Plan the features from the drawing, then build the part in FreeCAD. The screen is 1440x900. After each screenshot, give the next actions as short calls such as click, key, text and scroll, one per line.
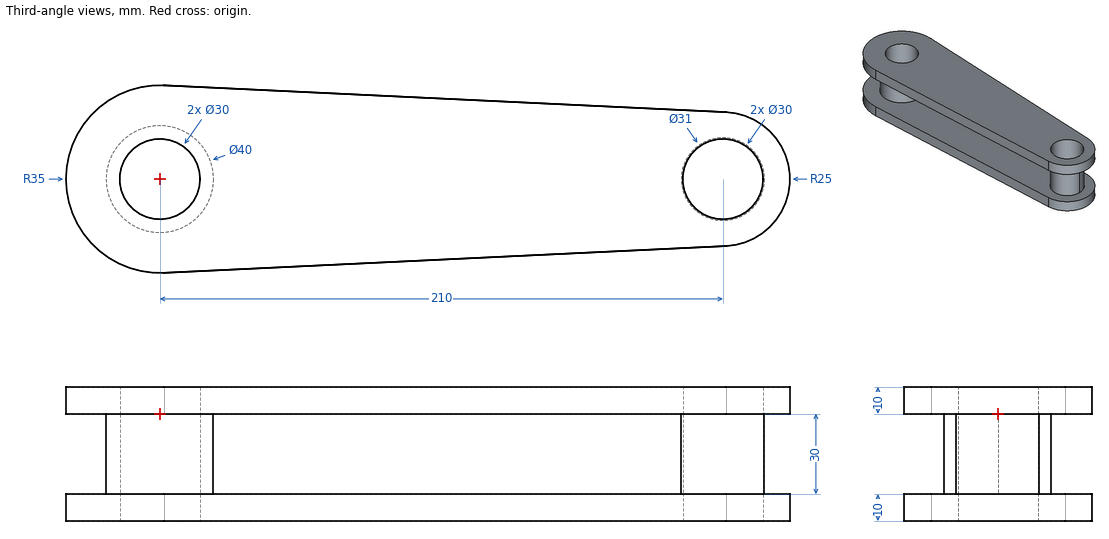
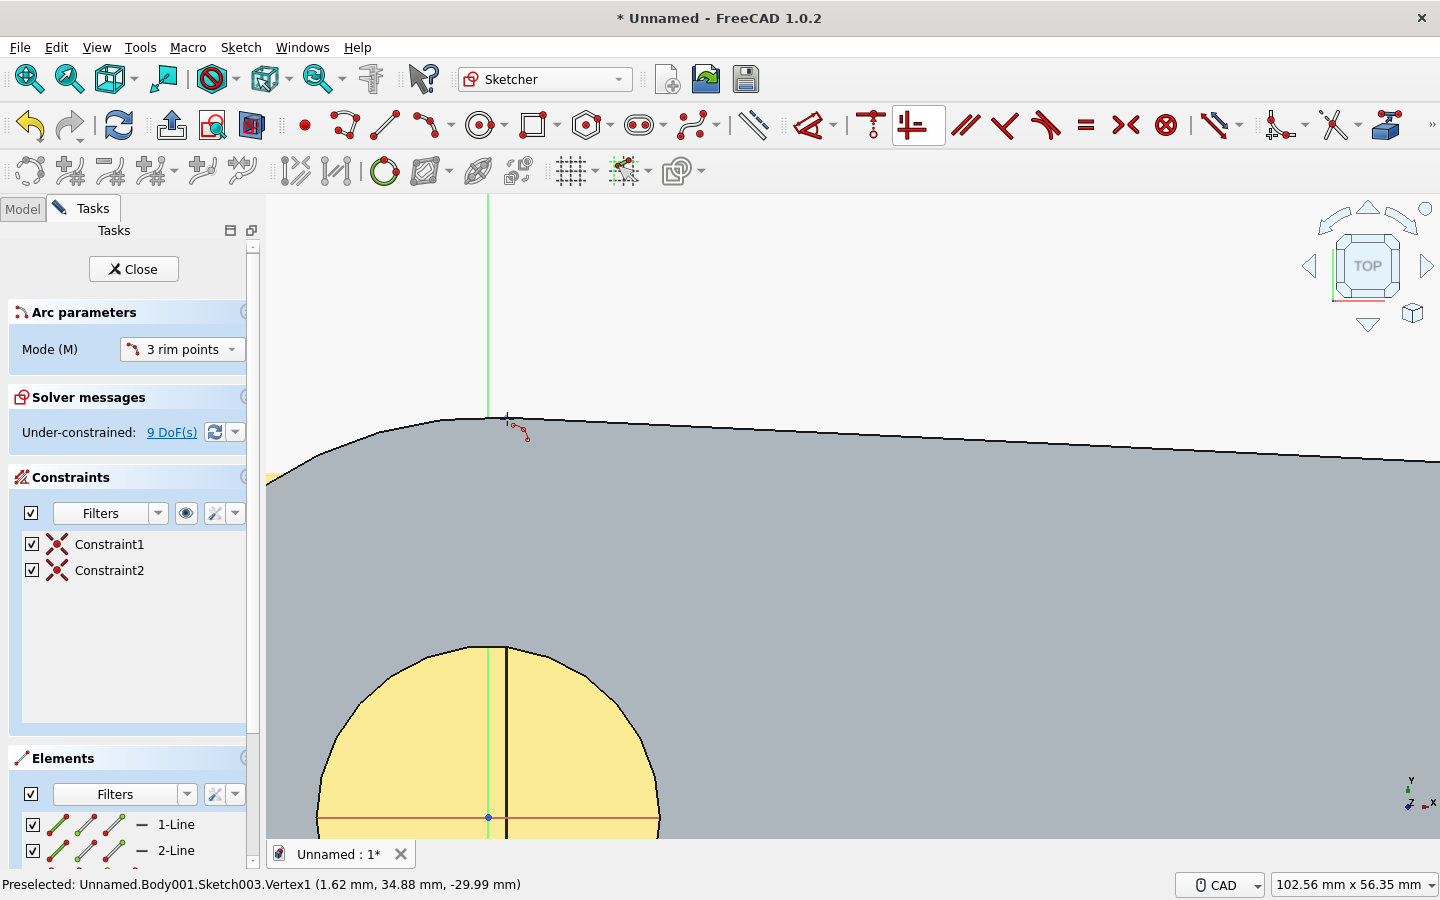
scroll(507, 418, down, 7)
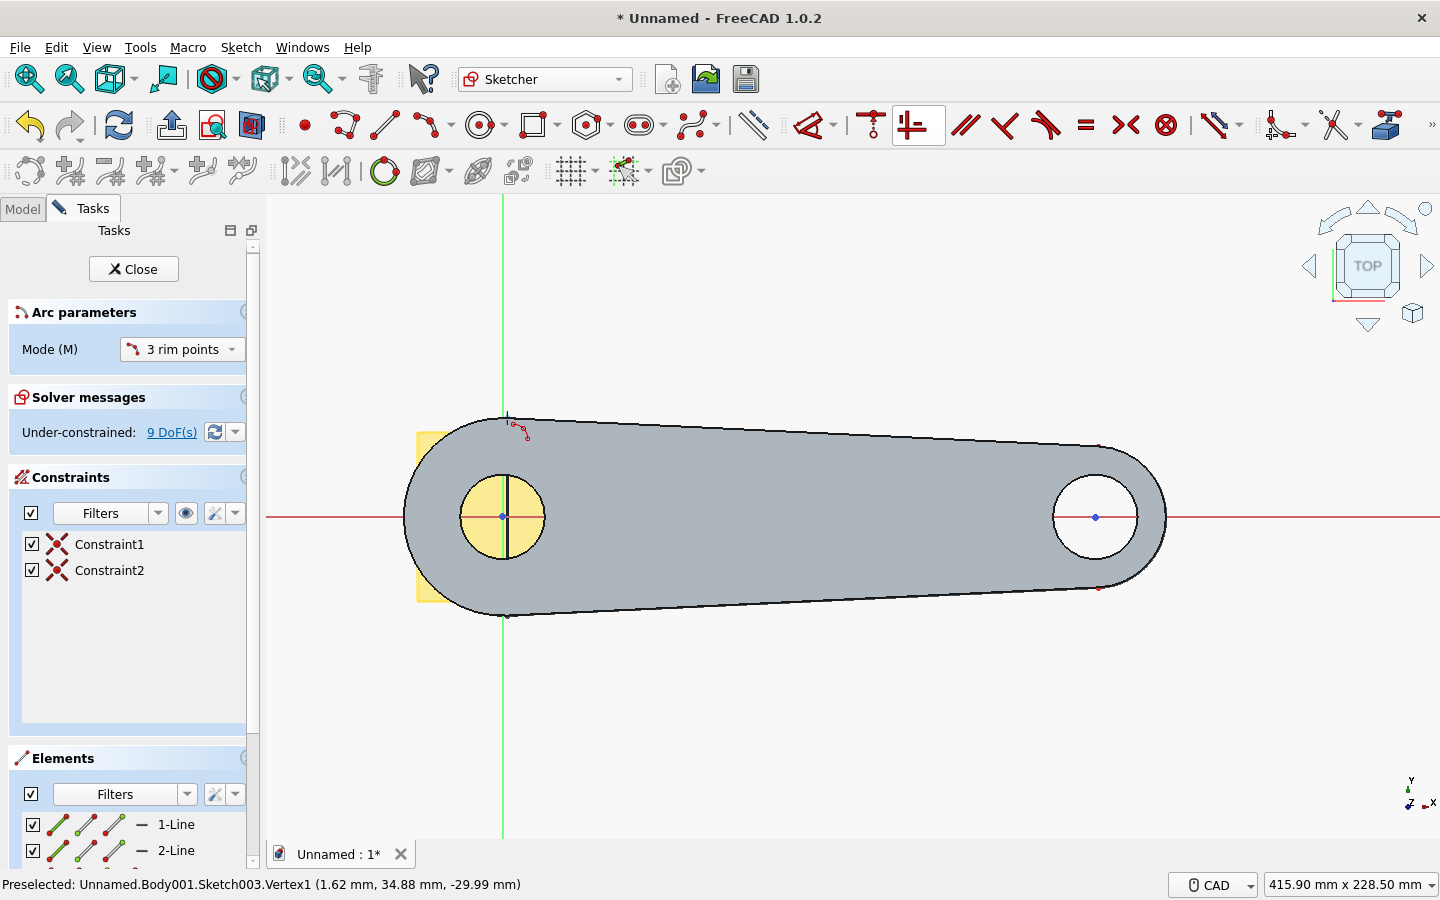
click(409, 485)
key(Escape)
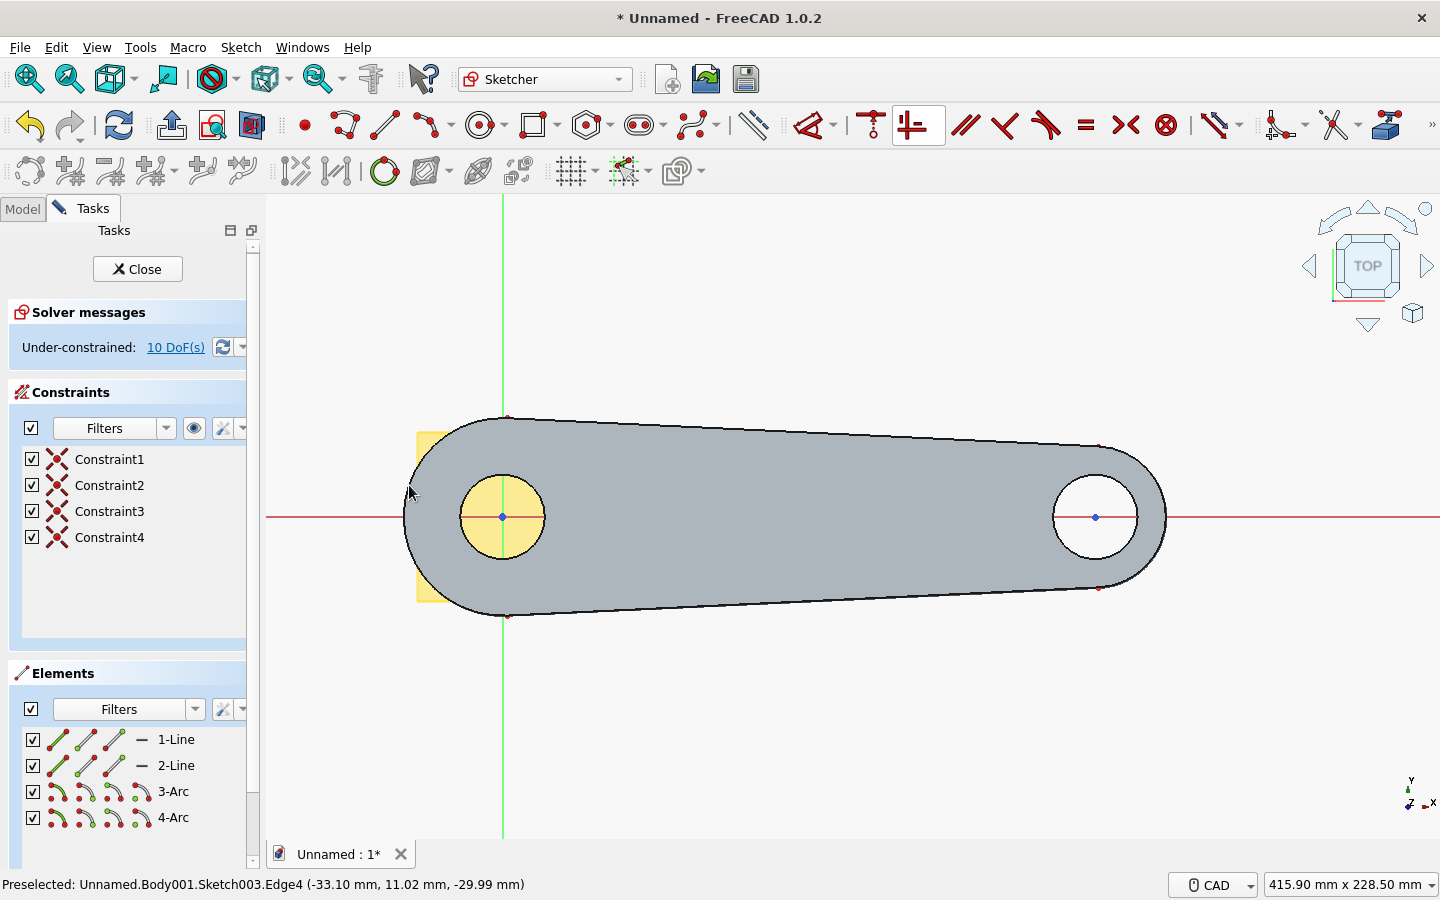
click(685, 427)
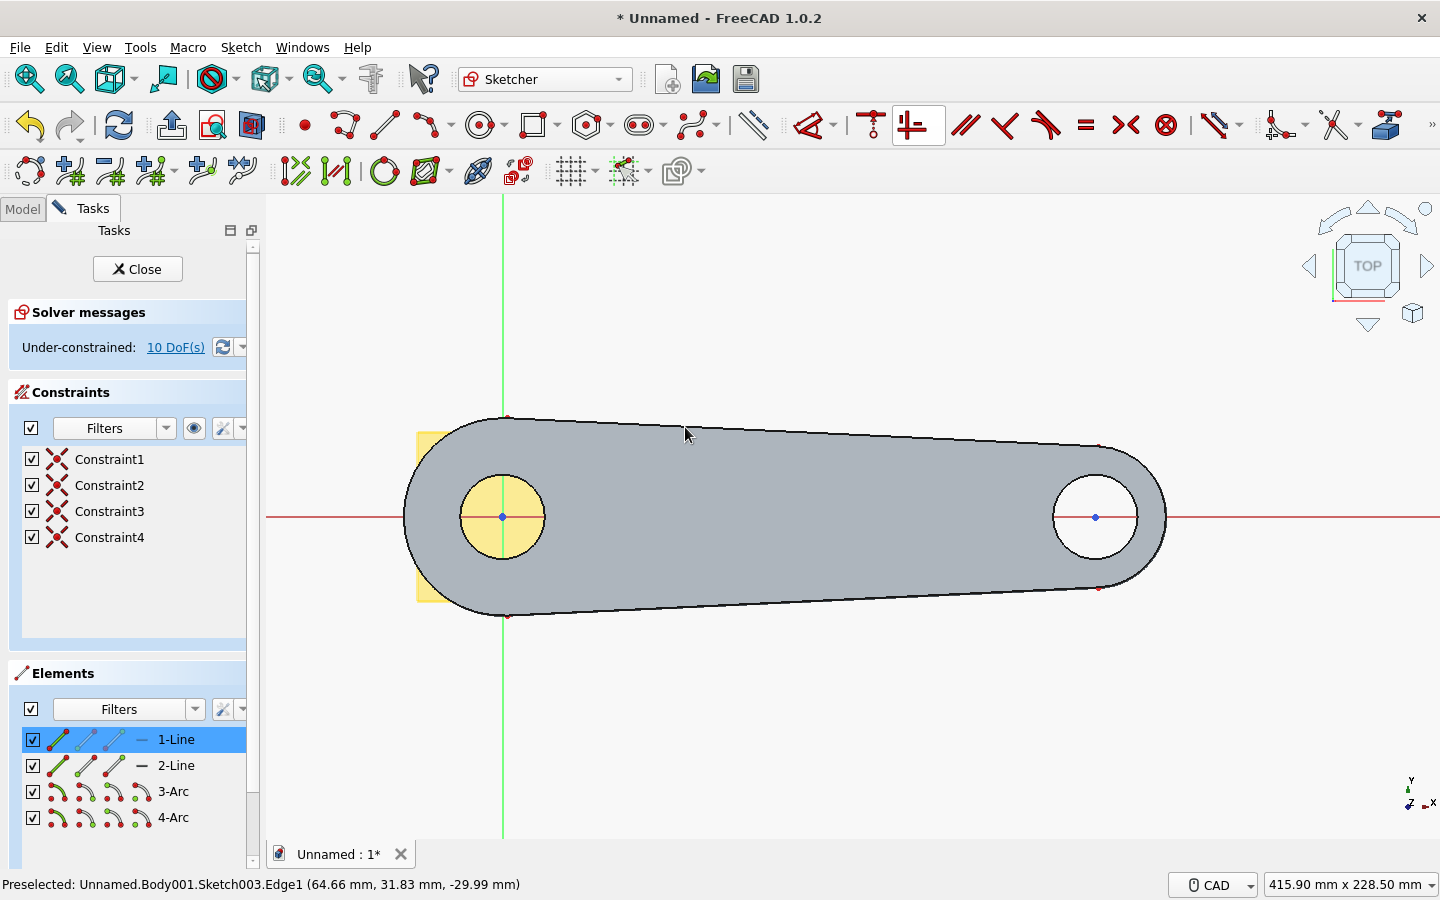
click(1154, 558)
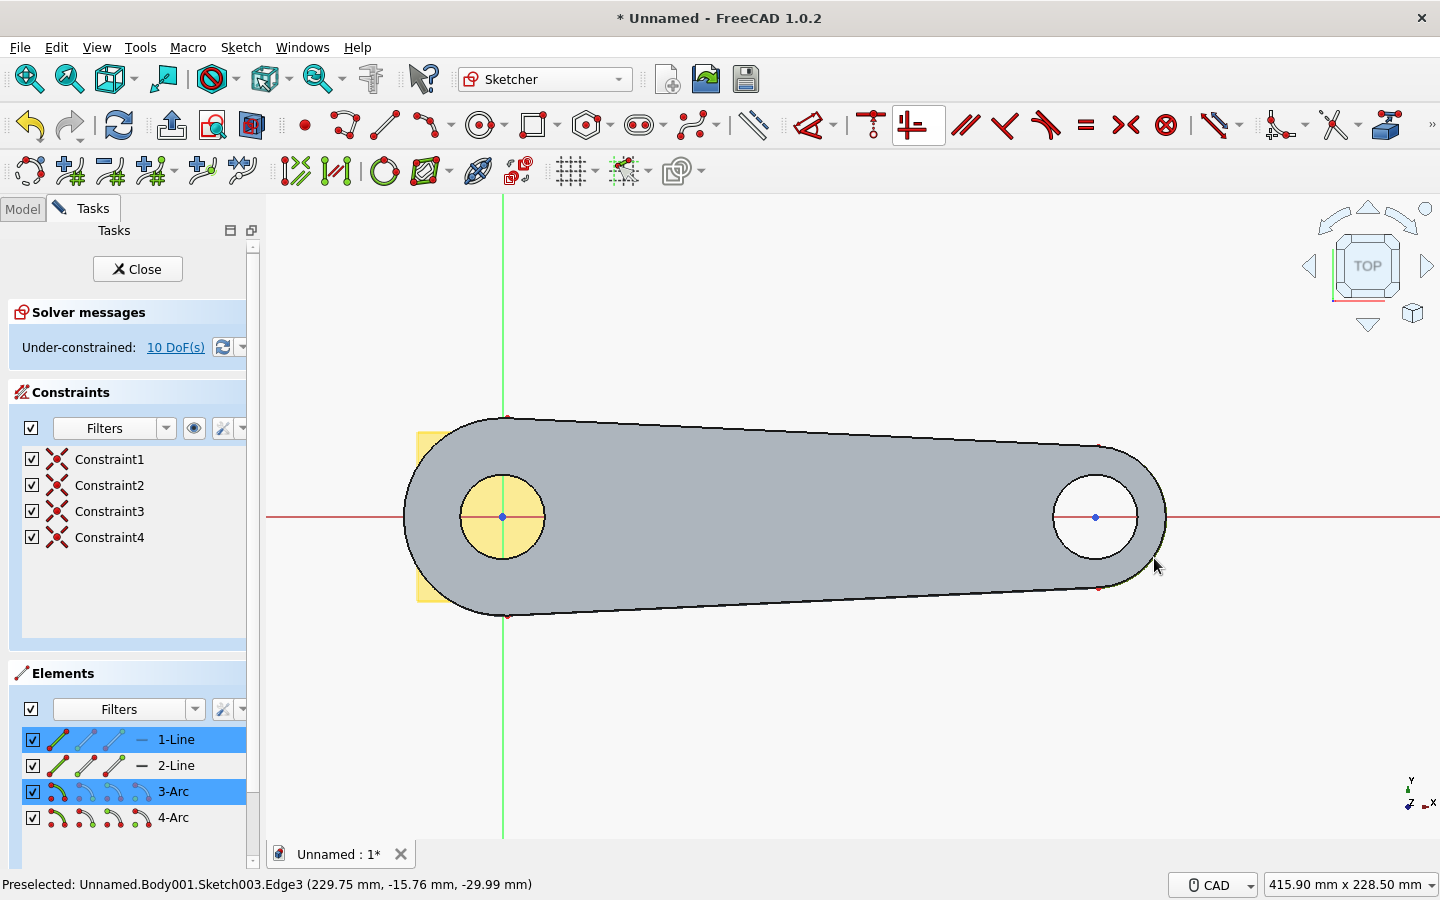
key(t)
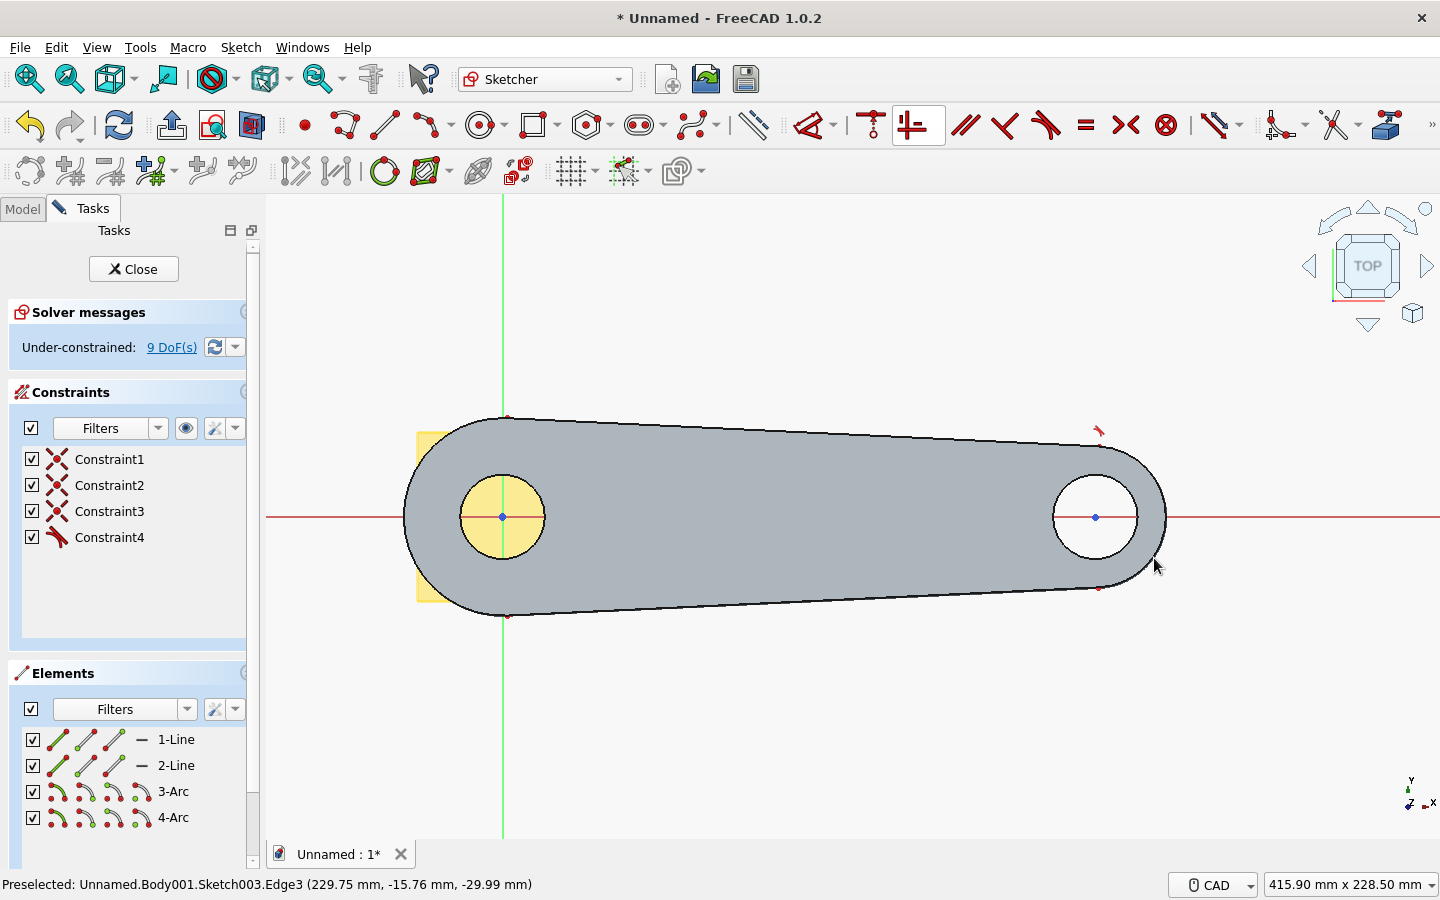
click(685, 427)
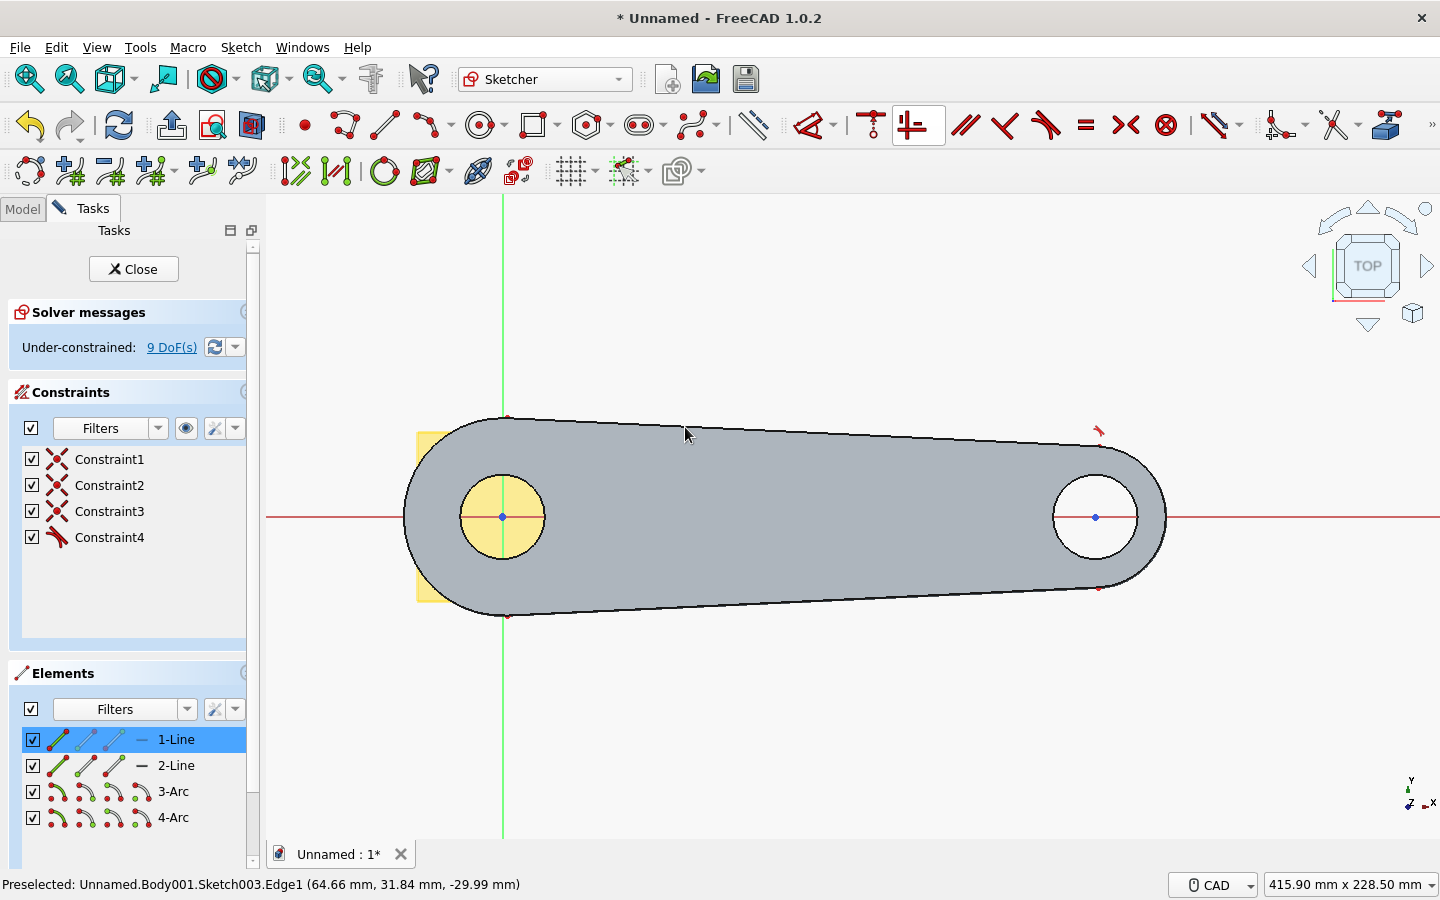
click(424, 458)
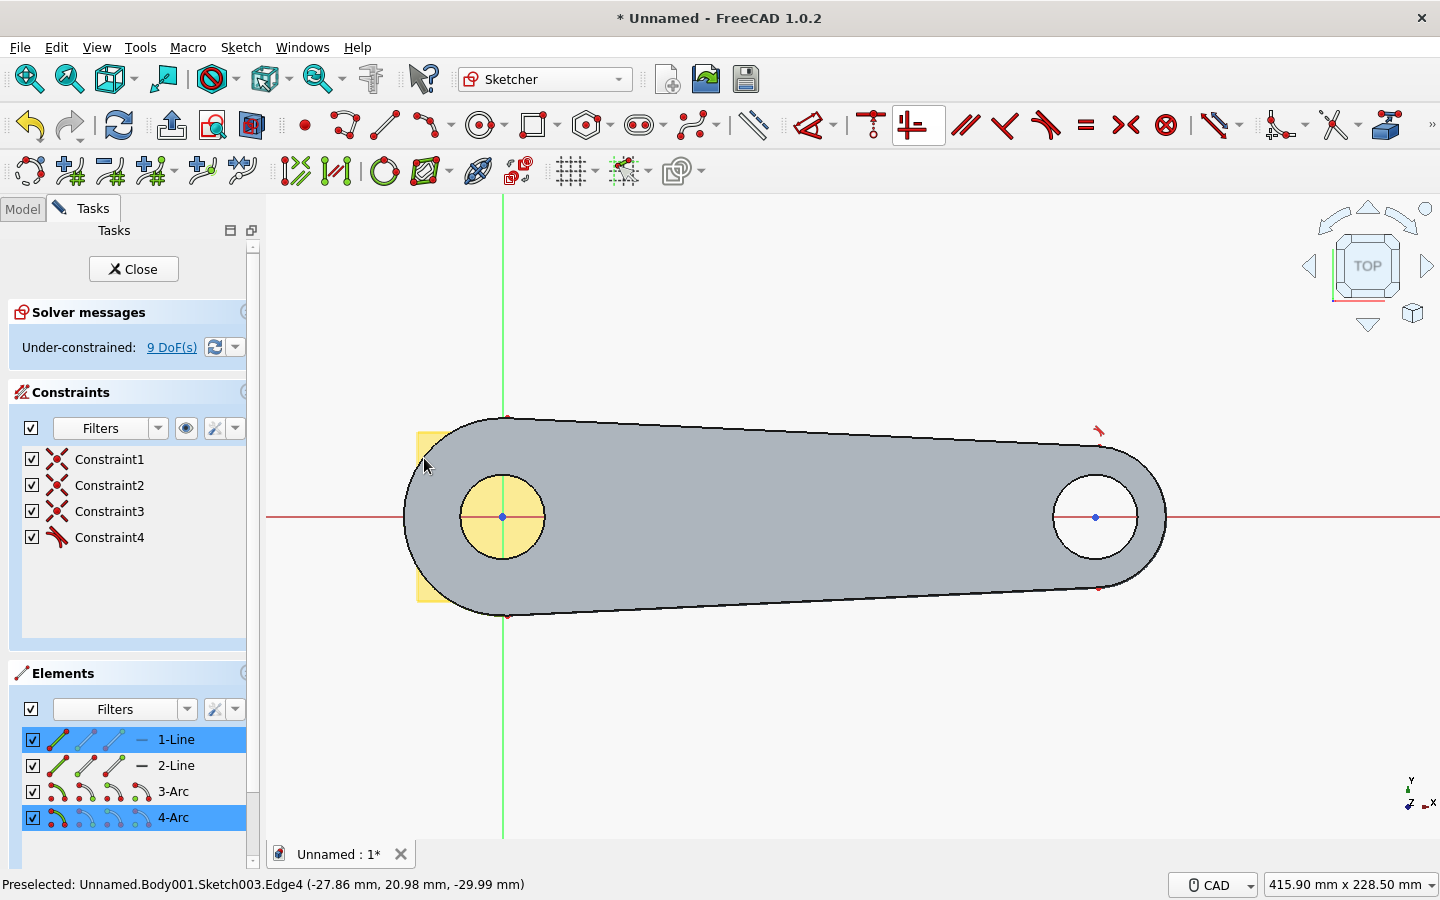
key(t)